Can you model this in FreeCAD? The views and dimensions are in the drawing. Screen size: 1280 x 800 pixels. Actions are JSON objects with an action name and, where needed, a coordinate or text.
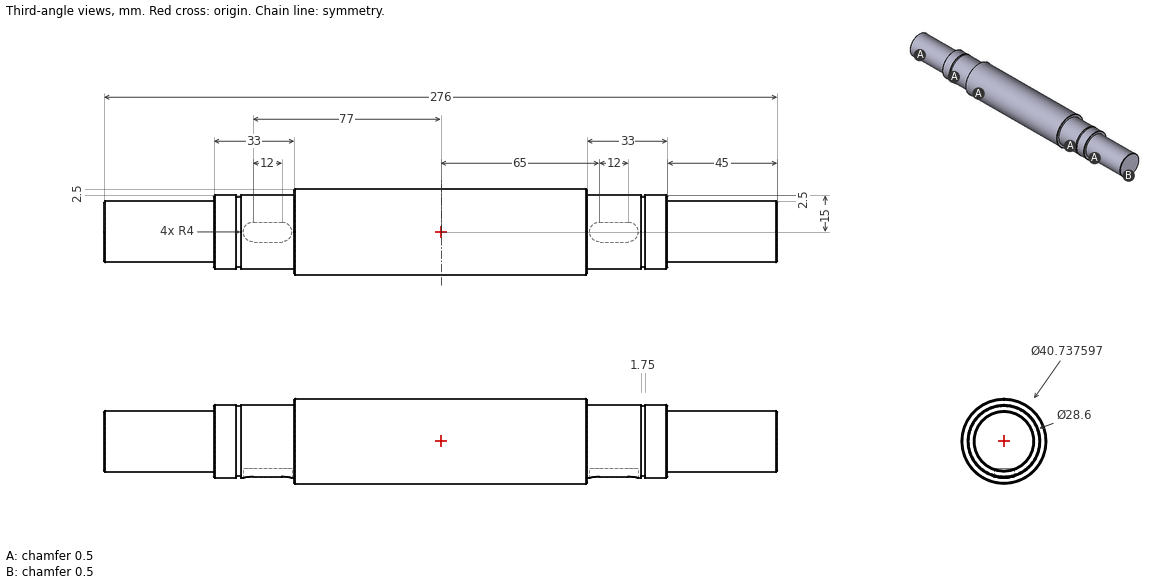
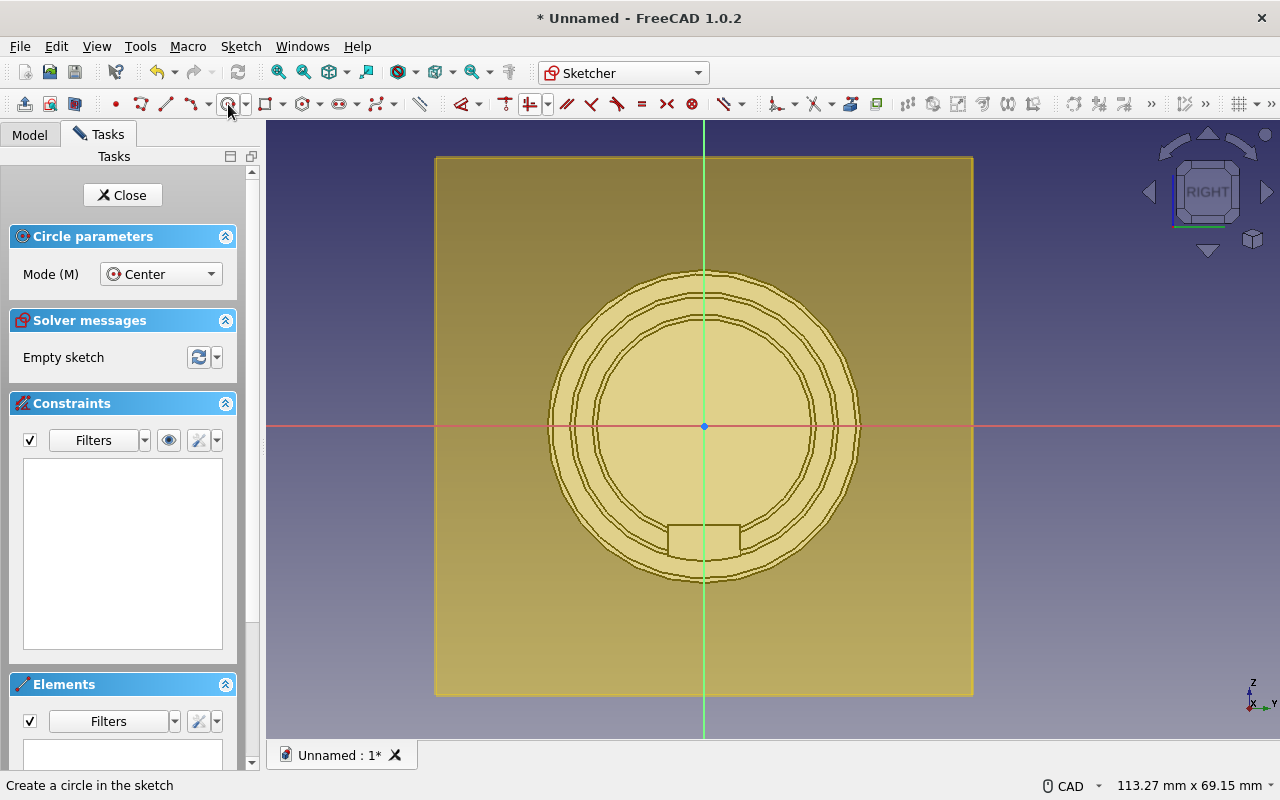
{"action": "left_click", "coordinate": [704, 426]}
{"action": "mouse_move", "coordinate": [833, 298]}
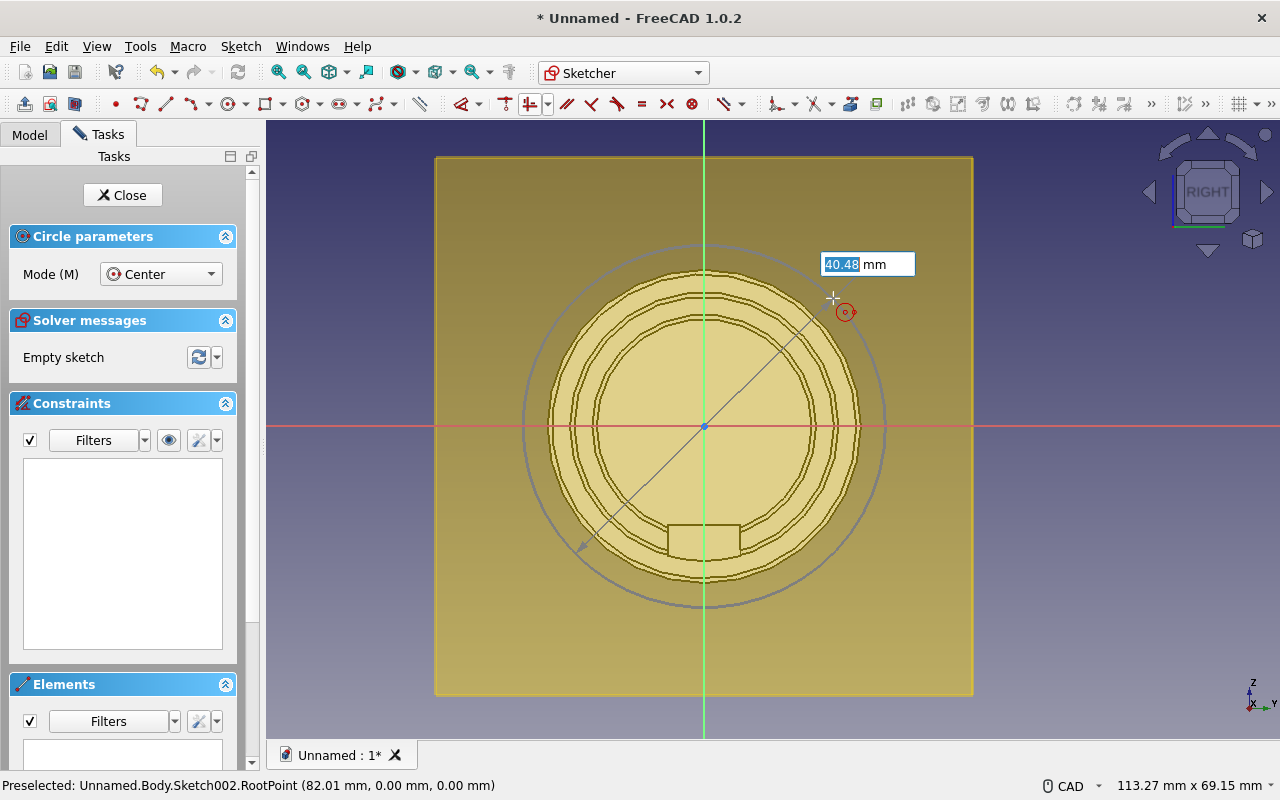
{"action": "type", "text": "40.737597"}
{"action": "key", "text": "Return"}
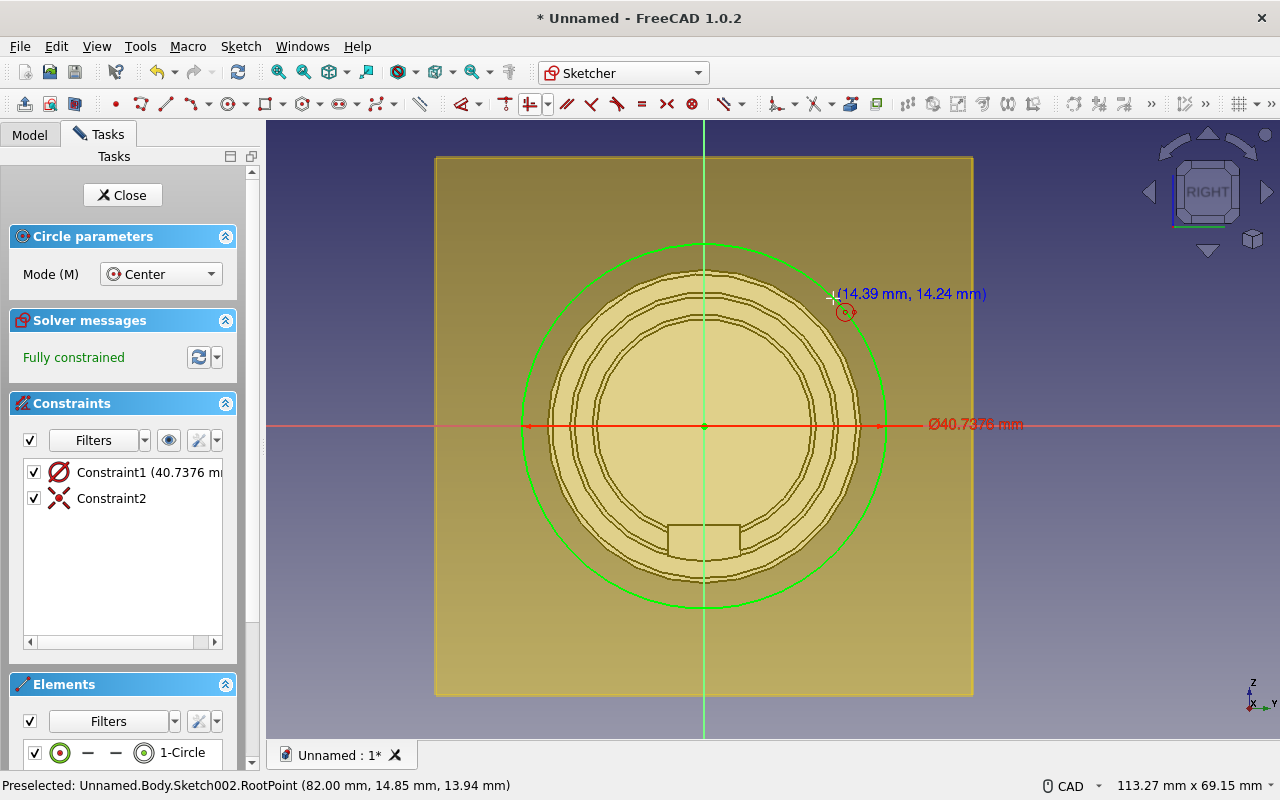
{"action": "left_click", "coordinate": [704, 426]}
{"action": "mouse_move", "coordinate": [795, 336]}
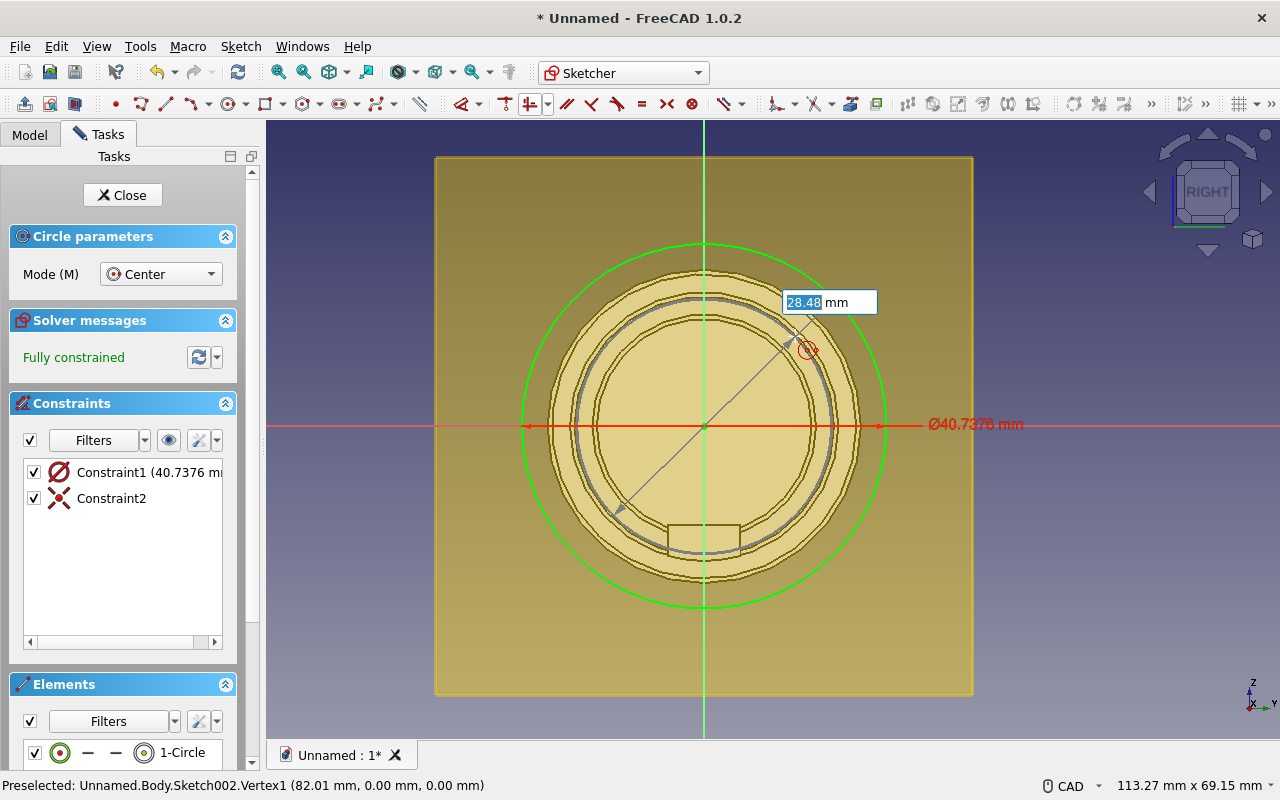
{"action": "type", "text": "28.6"}
{"action": "key", "text": "Return"}
{"action": "key", "text": "Escape"}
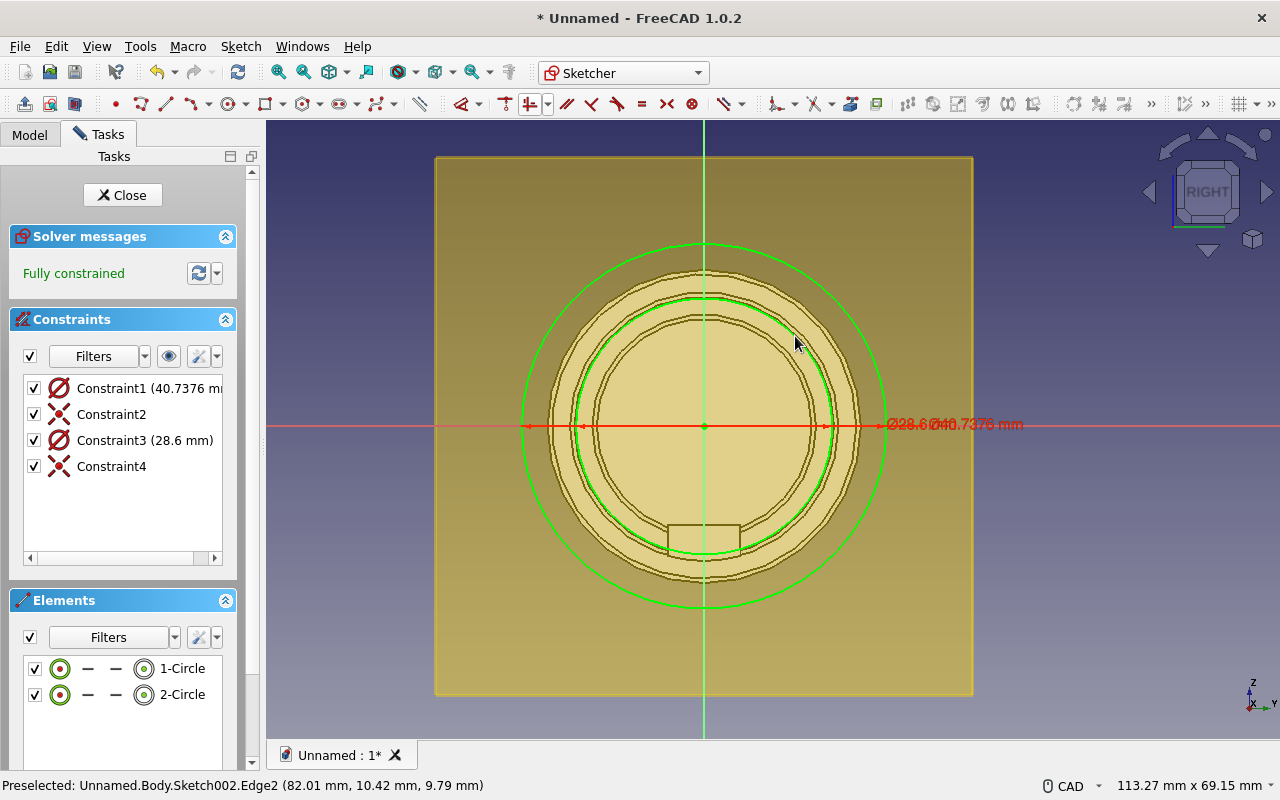
{"action": "left_click", "coordinate": [123, 195]}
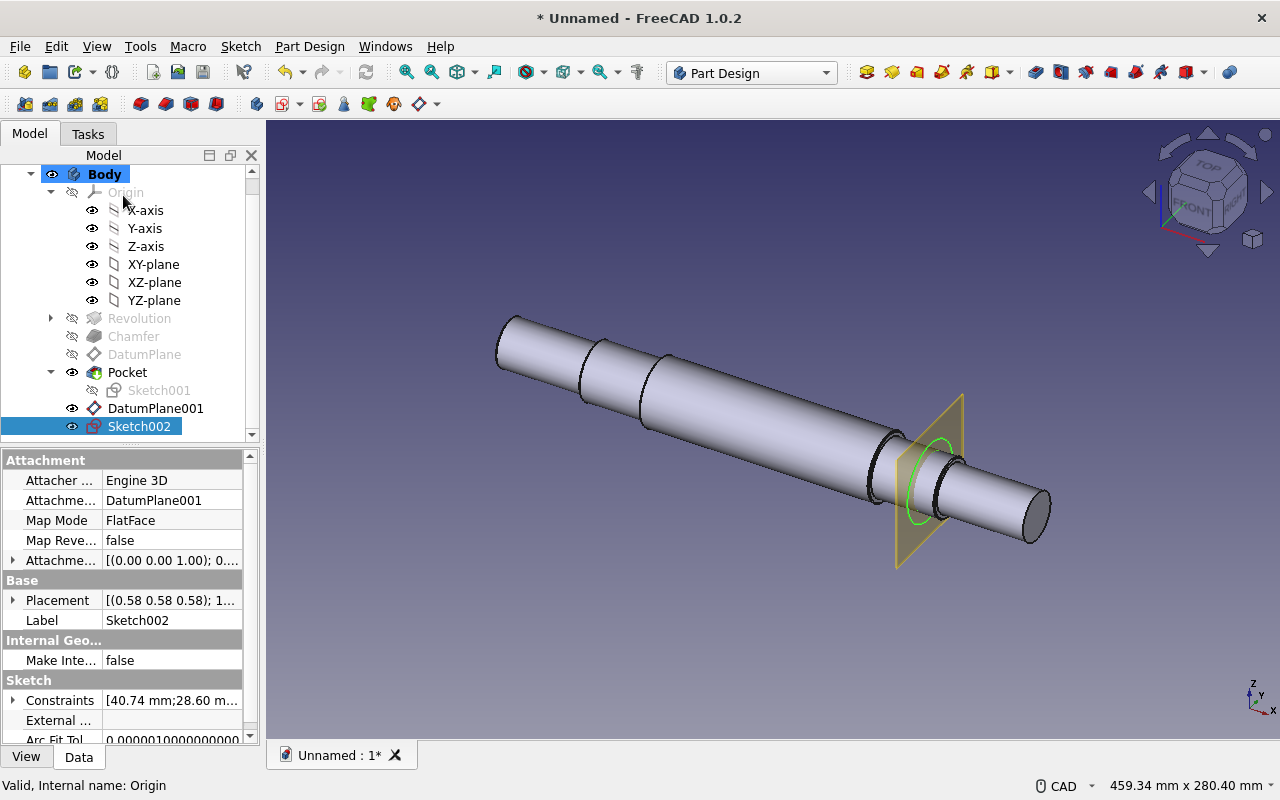
{"action": "left_click", "coordinate": [1036, 72]}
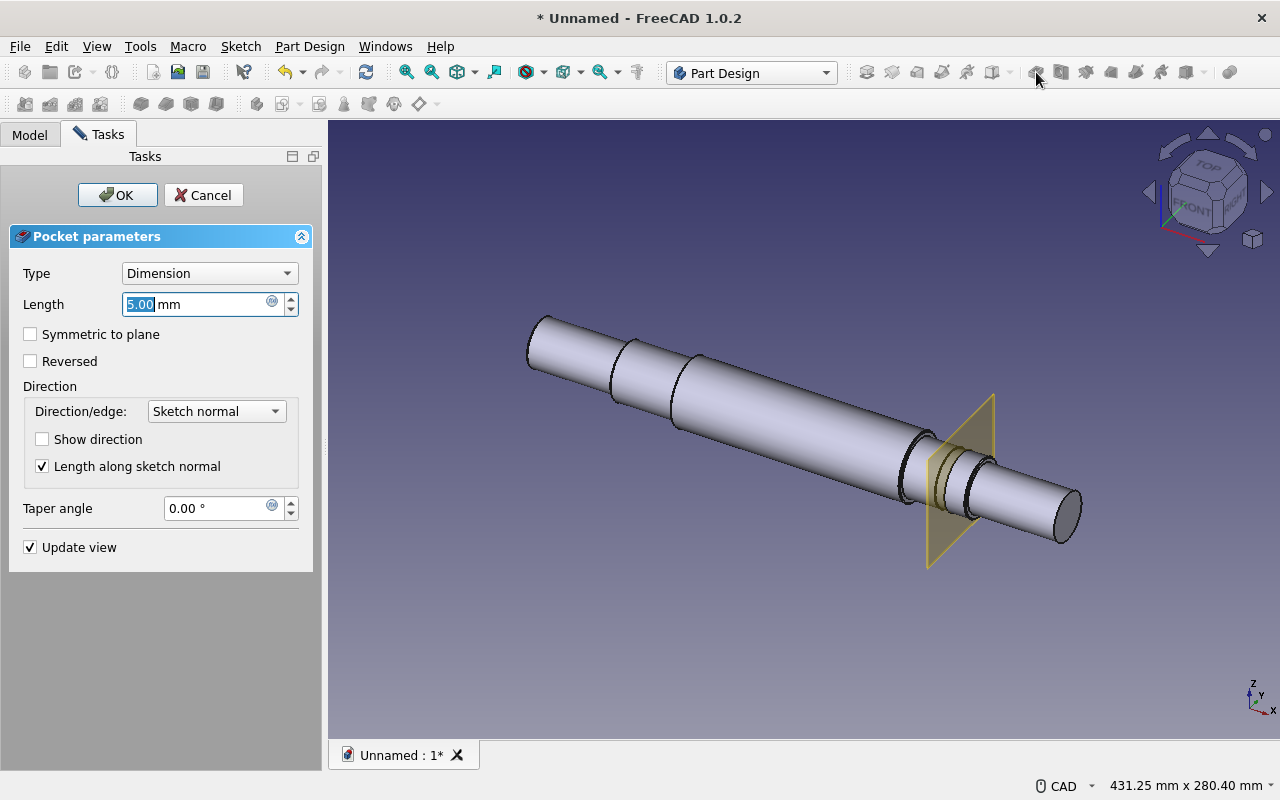
{"action": "type", "text": "1.75"}
{"action": "key", "text": "Tab"}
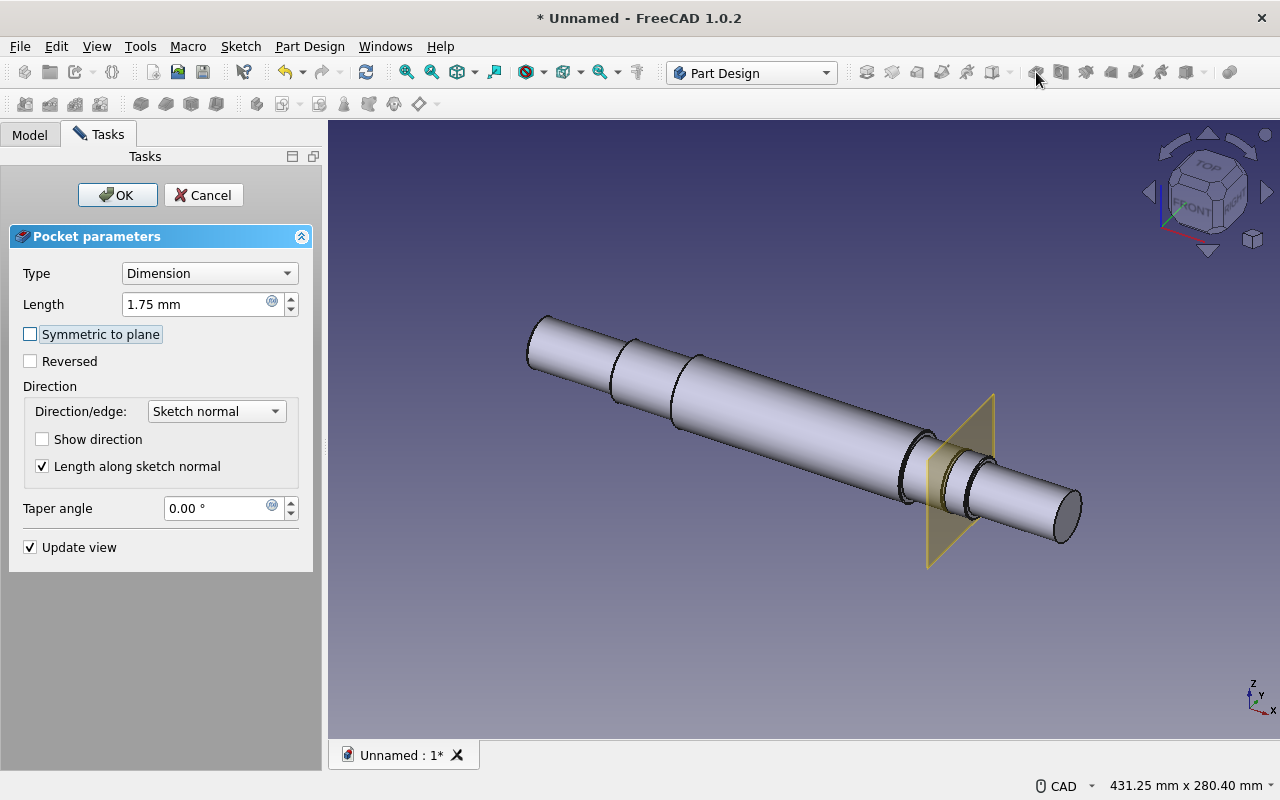
{"action": "left_click", "coordinate": [31, 361]}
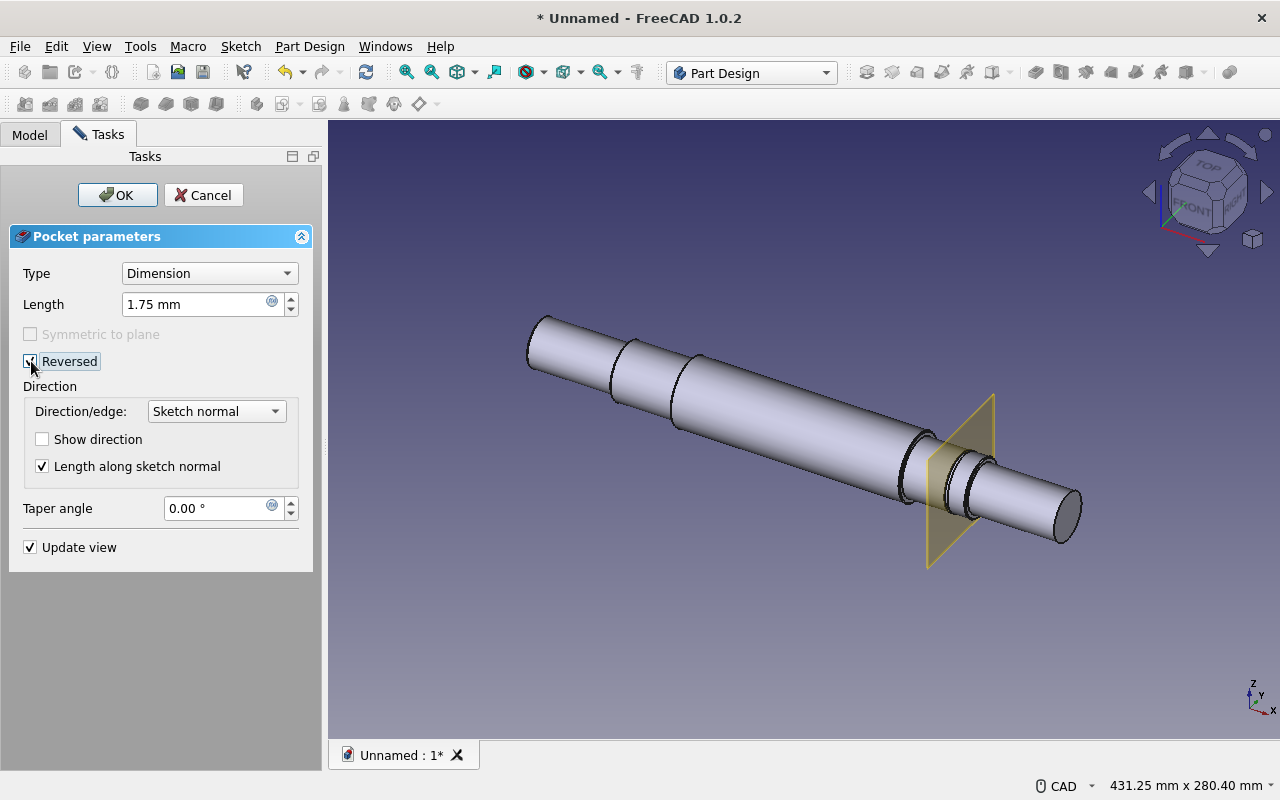
{"action": "left_click", "coordinate": [118, 195]}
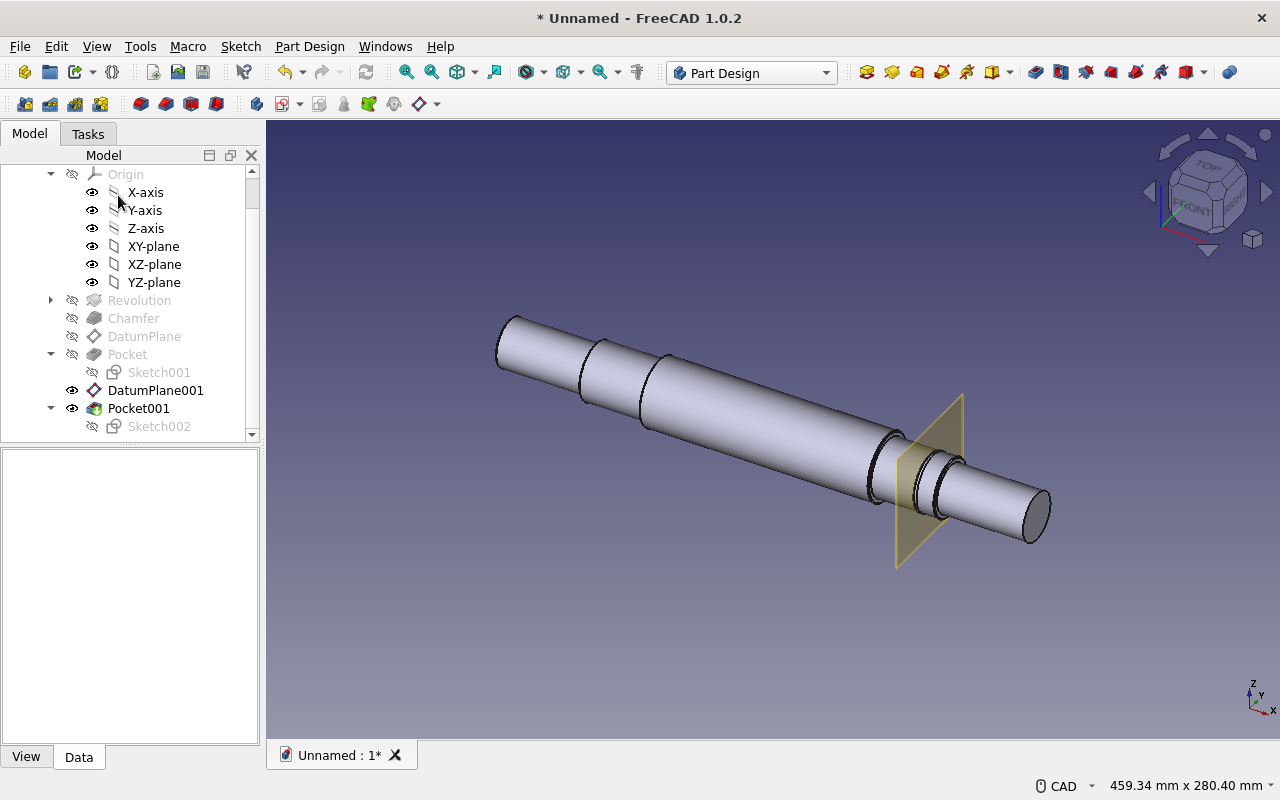
{"action": "left_click", "coordinate": [117, 390]}
{"action": "key", "text": "space"}